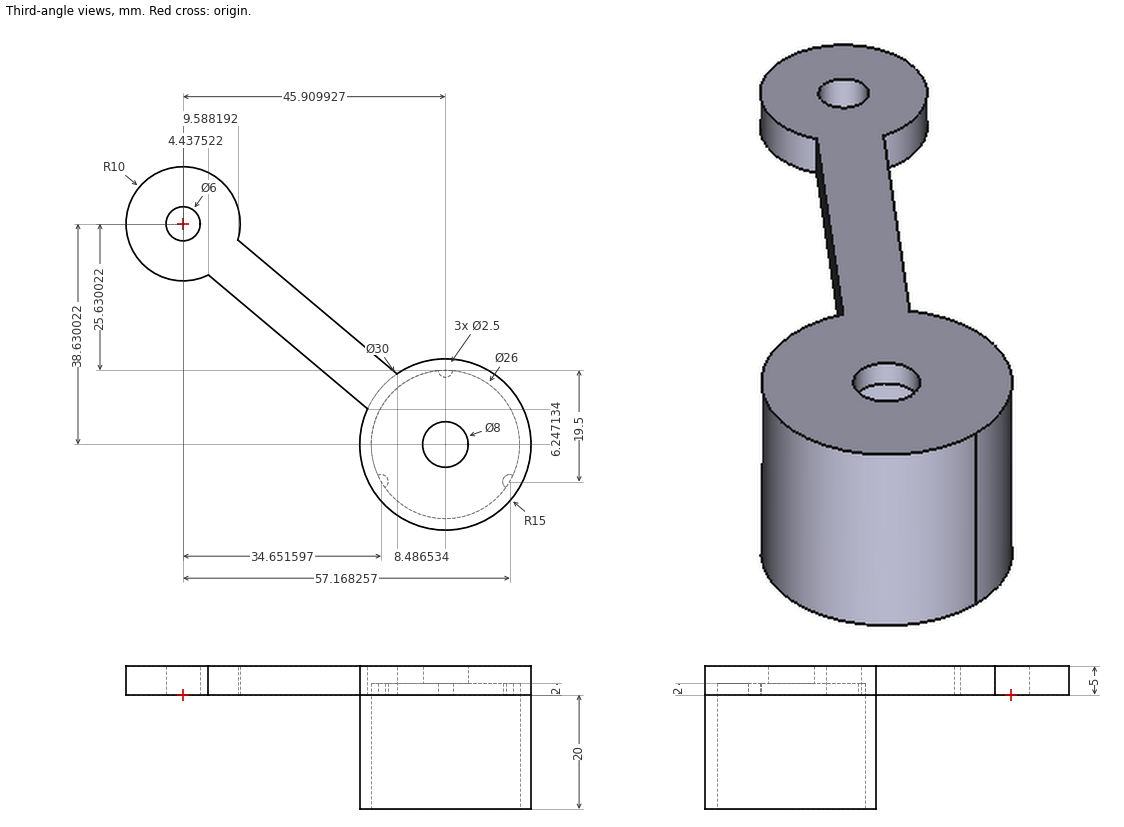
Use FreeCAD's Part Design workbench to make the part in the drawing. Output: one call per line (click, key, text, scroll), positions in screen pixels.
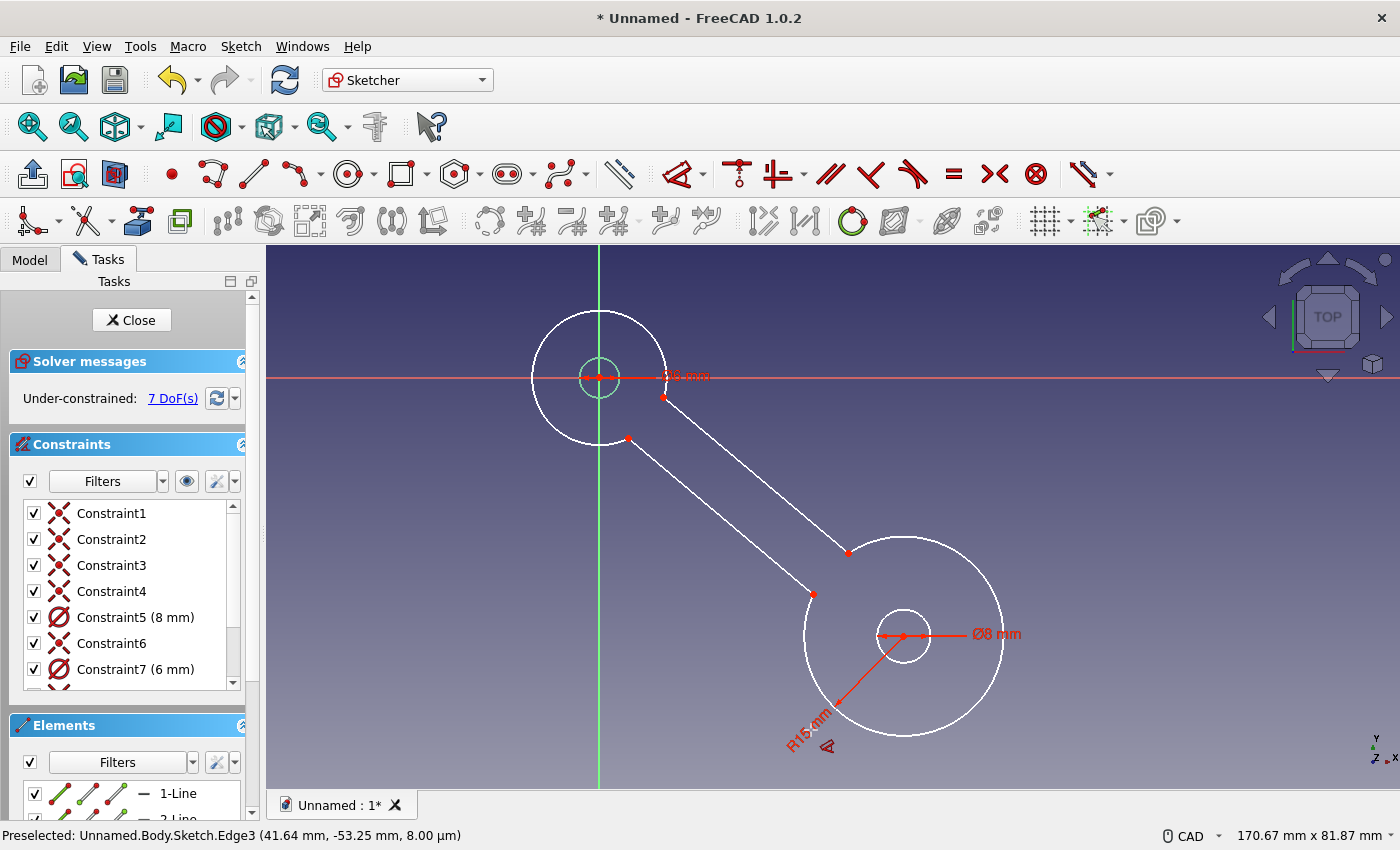
click(615, 312)
click(622, 281)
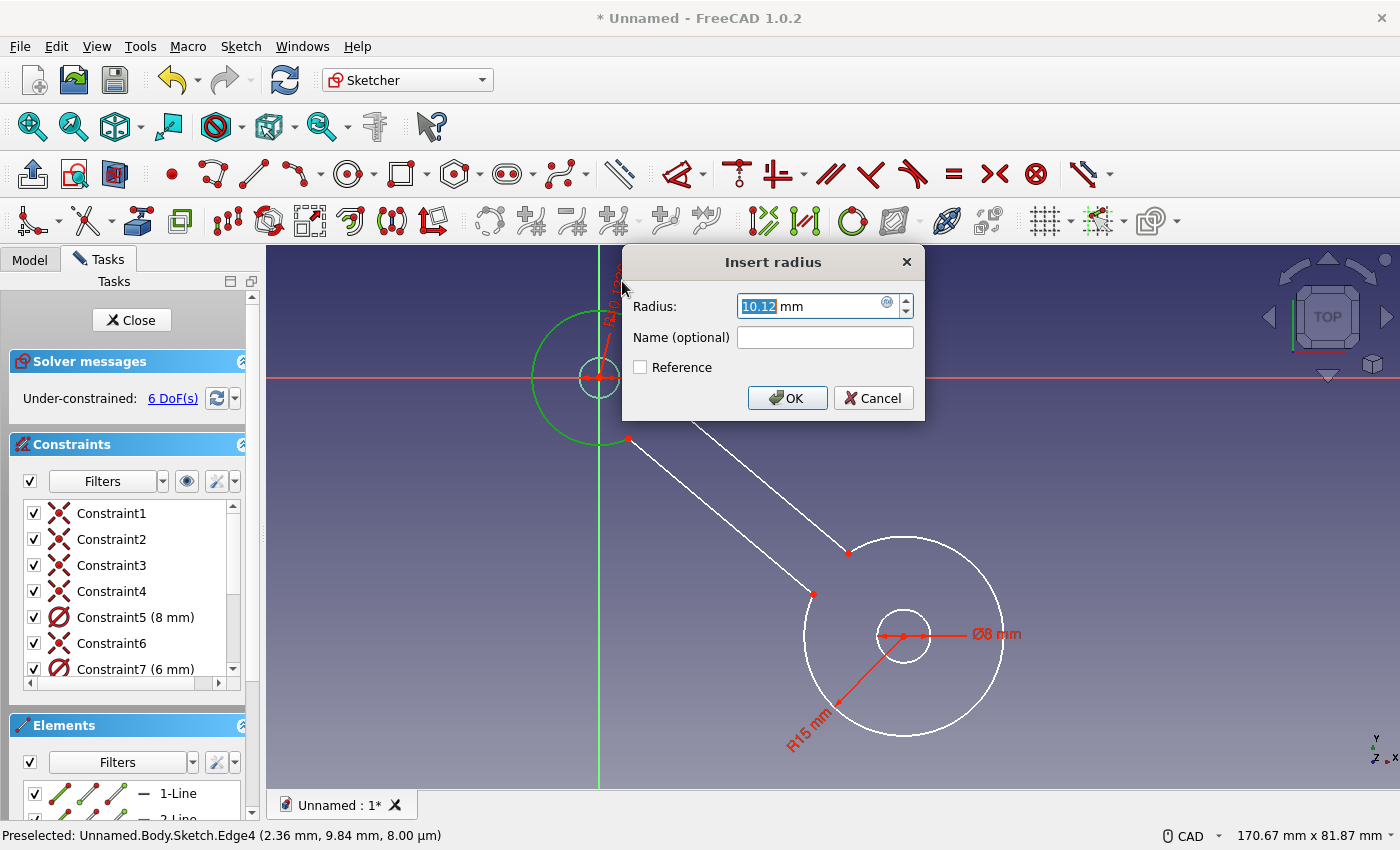
text(10)
key(Return)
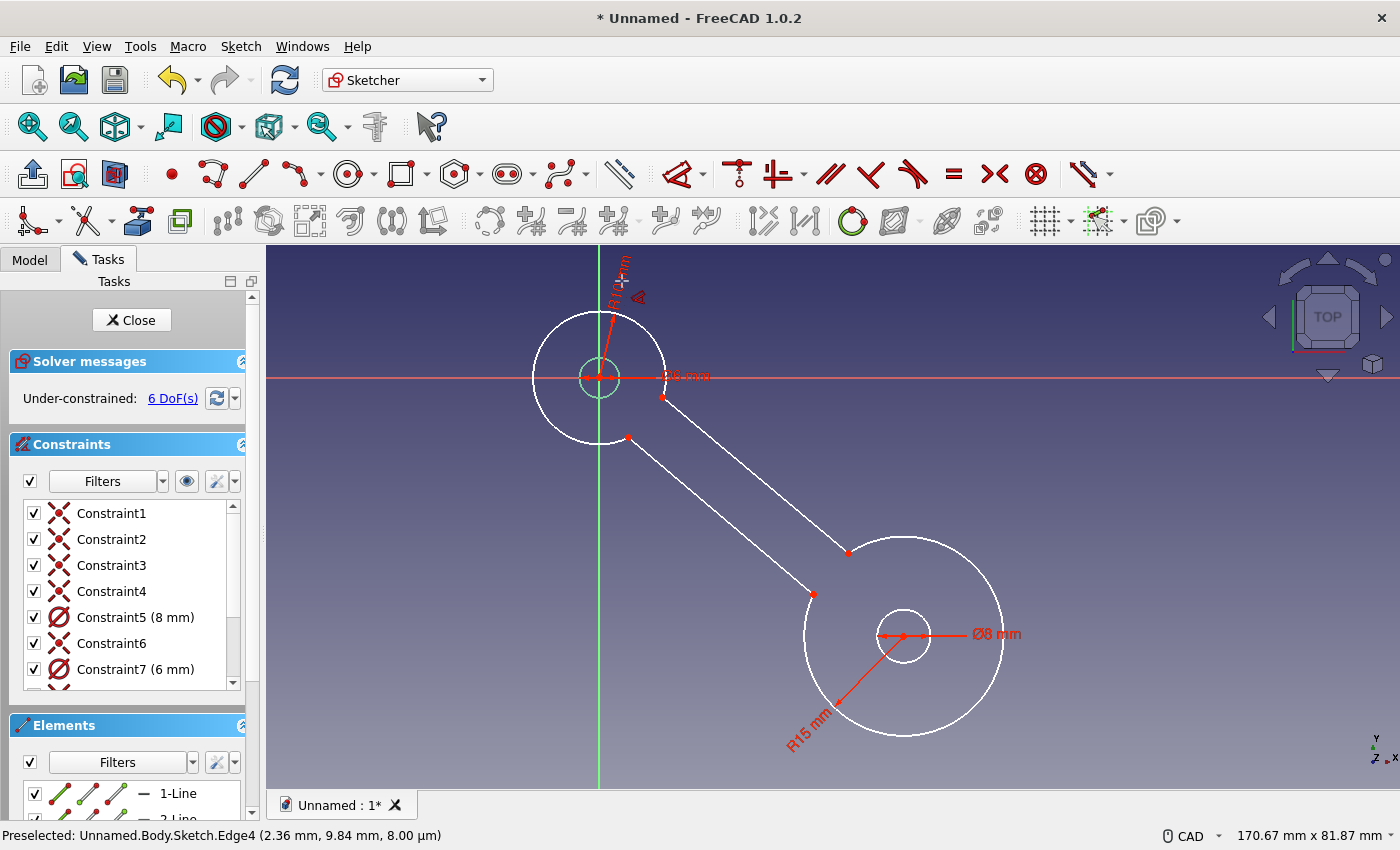
scroll(629, 438, up, 2)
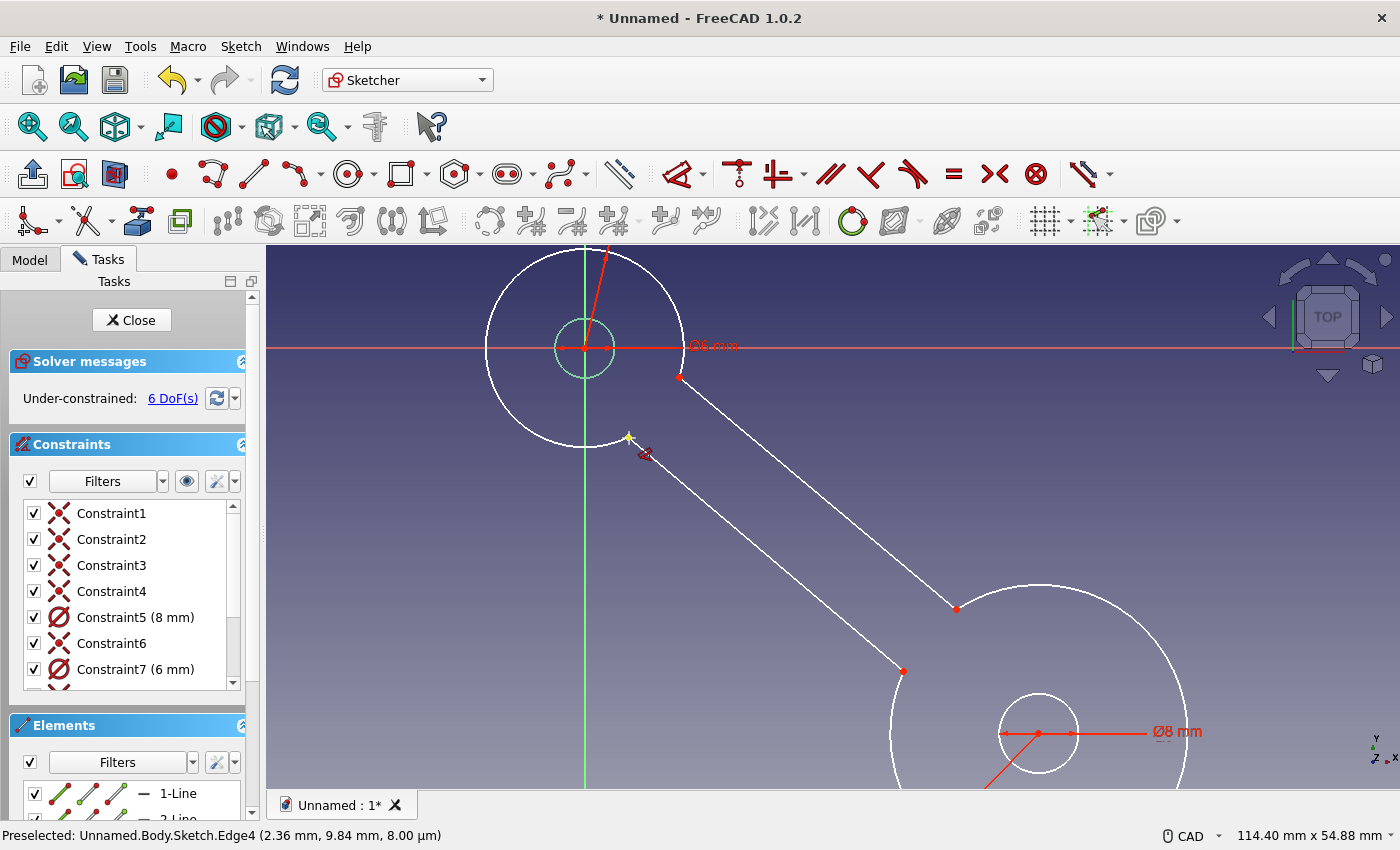
click(628, 437)
click(616, 314)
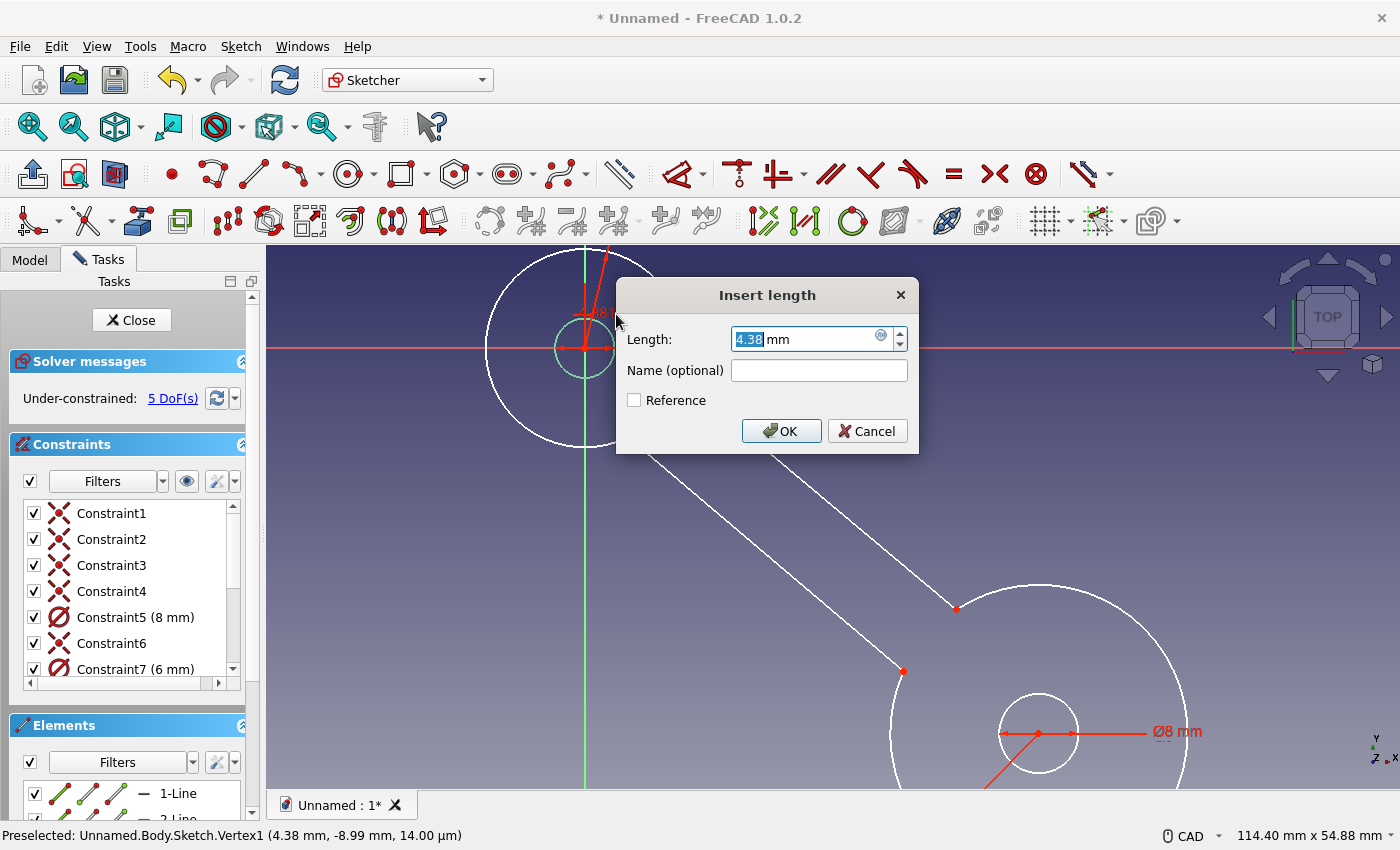
text(4.437522)
key(Return)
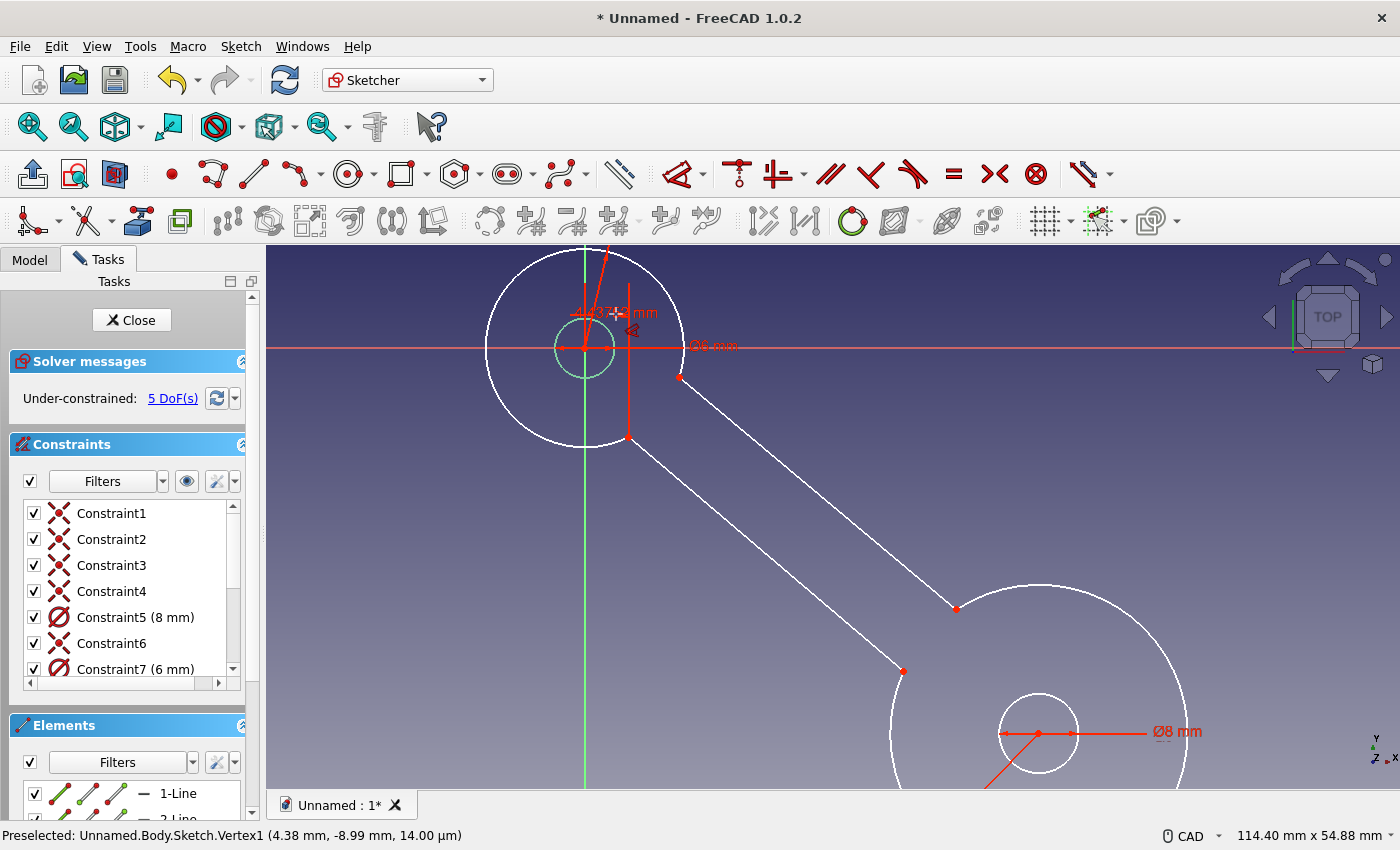
click(679, 377)
click(632, 411)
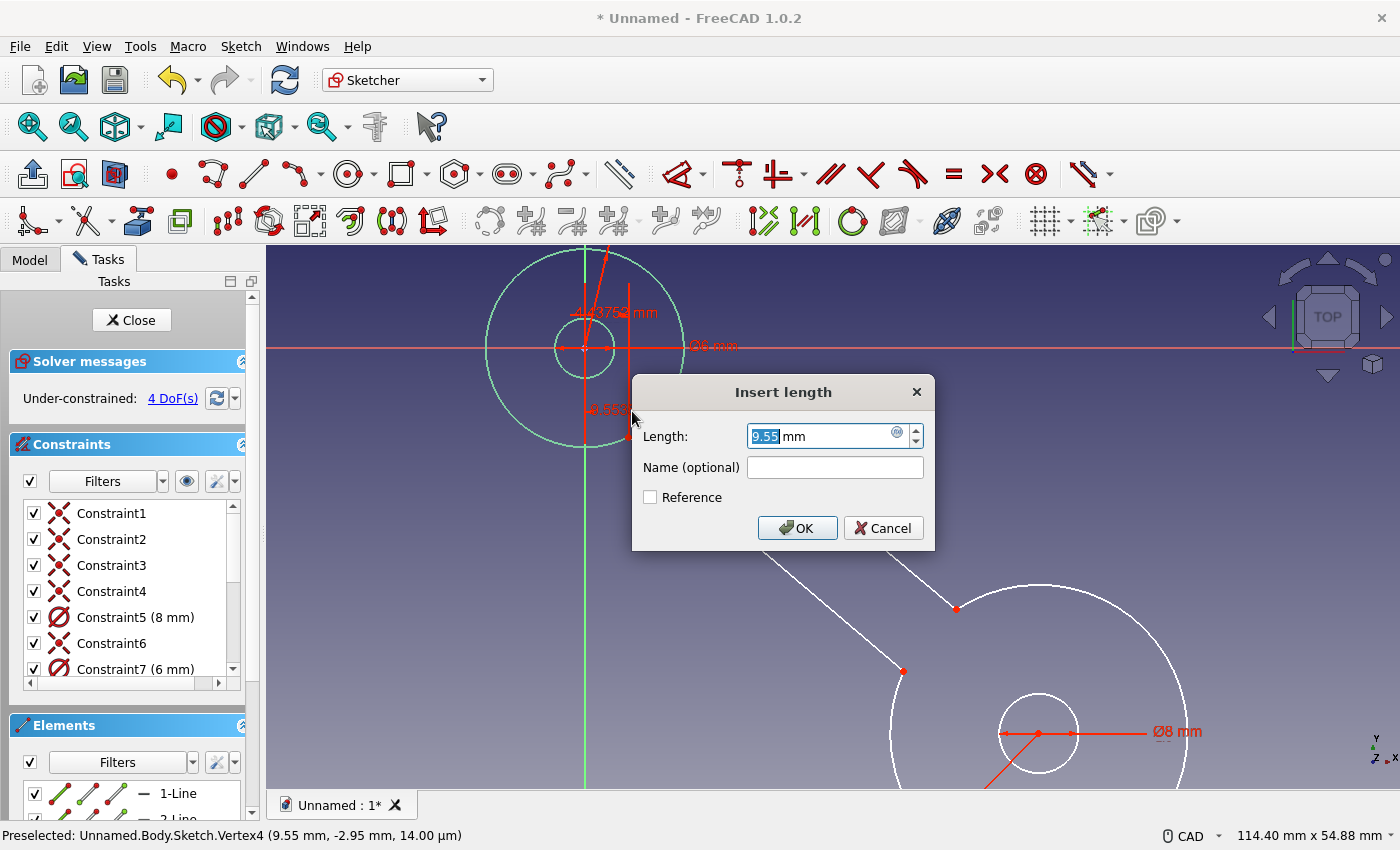
text(9.588192)
key(Return)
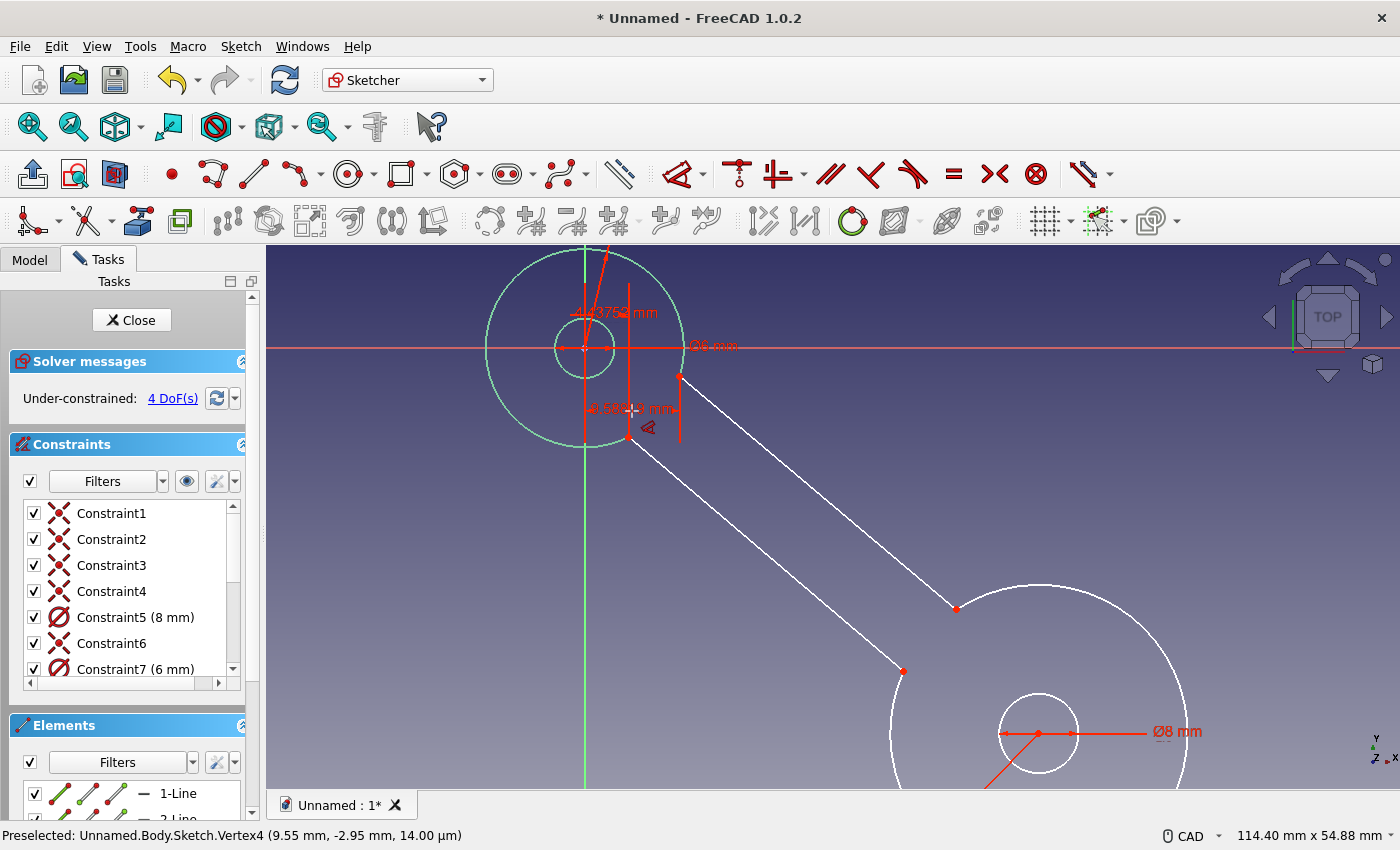
click(1039, 734)
click(812, 314)